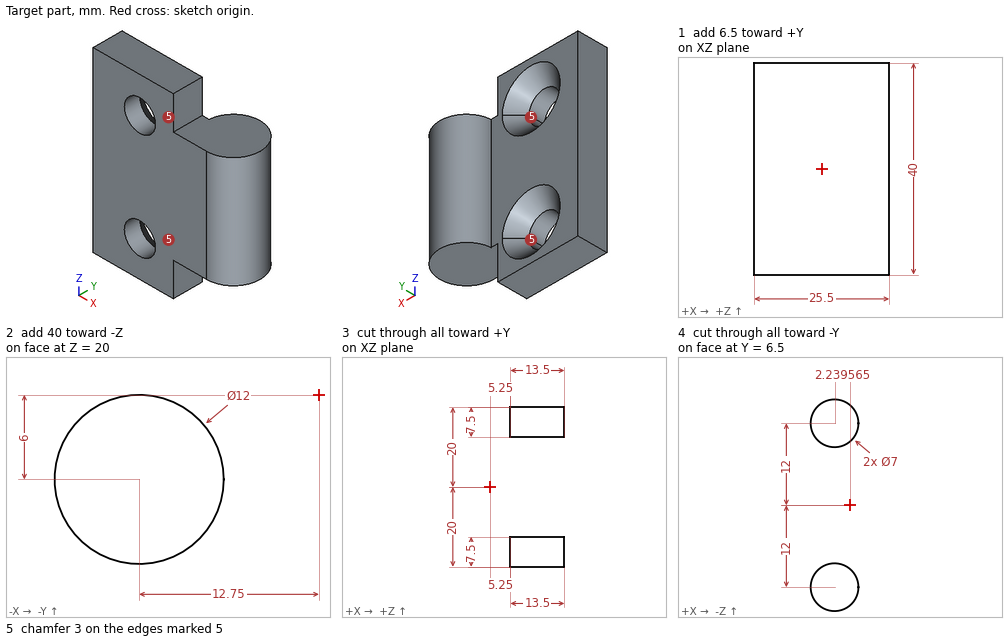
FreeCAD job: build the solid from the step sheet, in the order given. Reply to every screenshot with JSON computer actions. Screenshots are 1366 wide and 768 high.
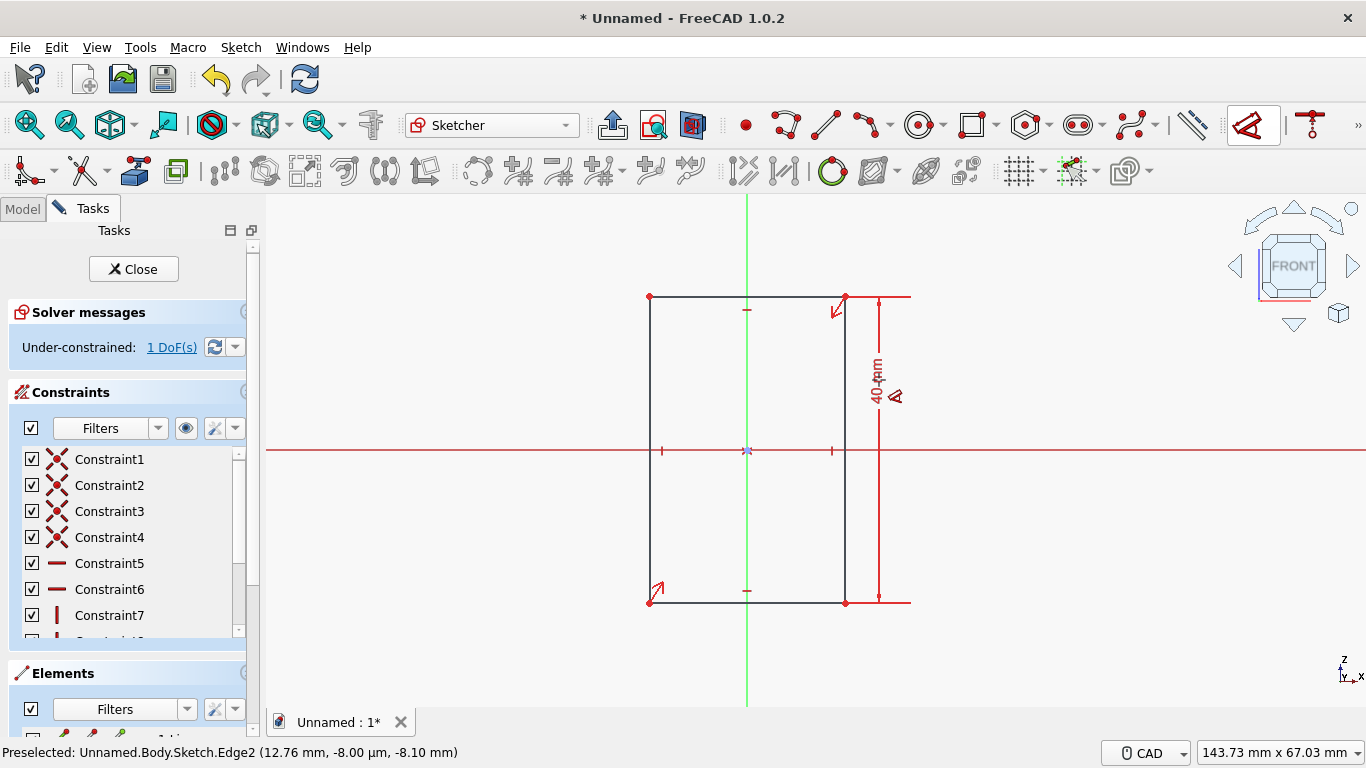
{"action": "left_click", "coordinate": [708, 603]}
{"action": "left_click", "coordinate": [702, 637]}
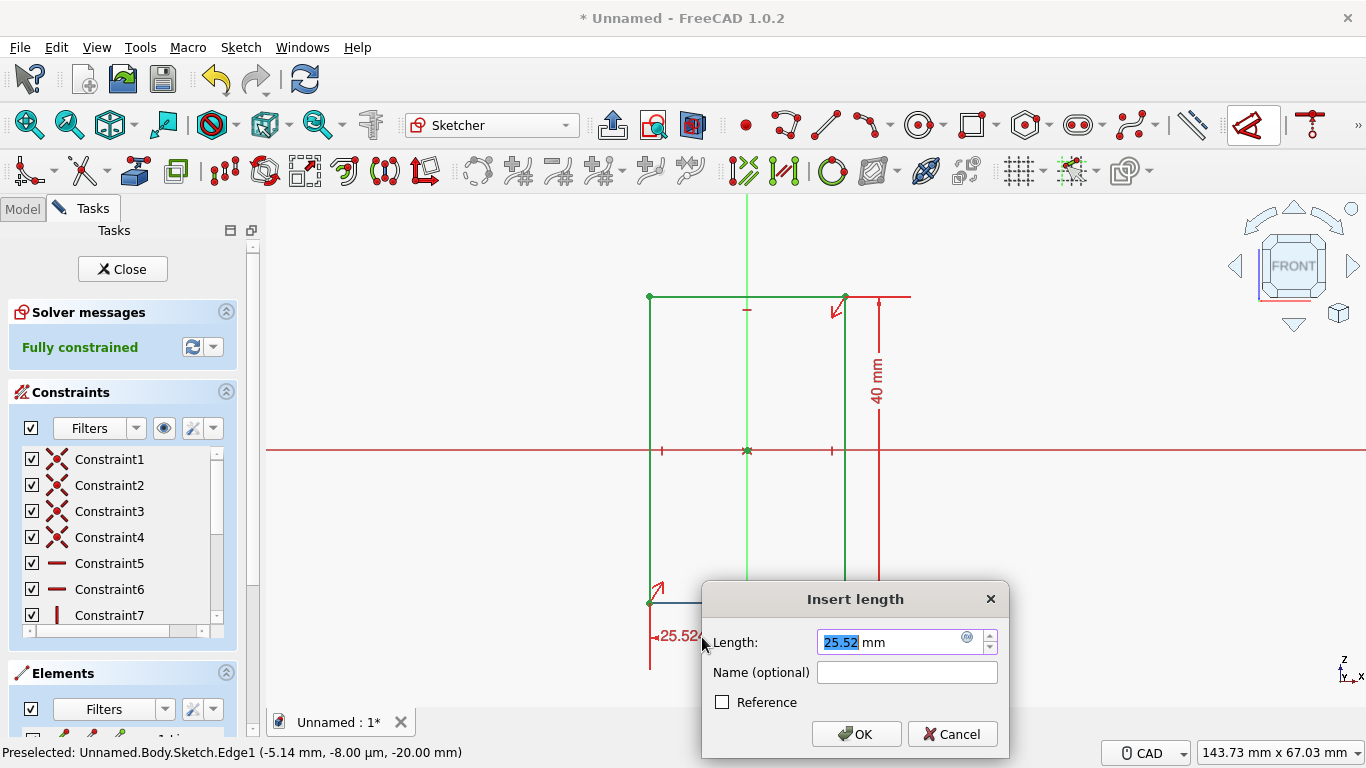
{"action": "type", "text": "25.5"}
{"action": "key", "text": "Return"}
{"action": "key", "text": "Escape"}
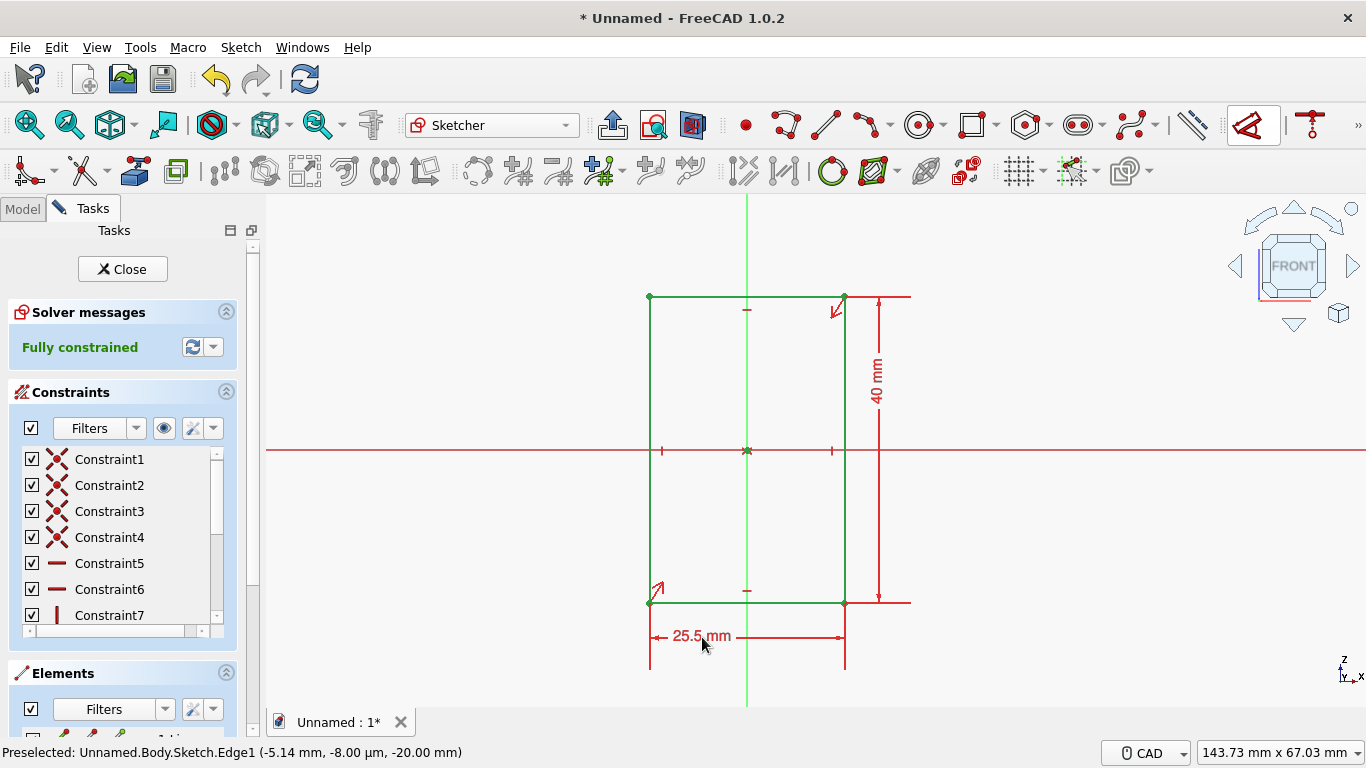
{"action": "left_click", "coordinate": [123, 269]}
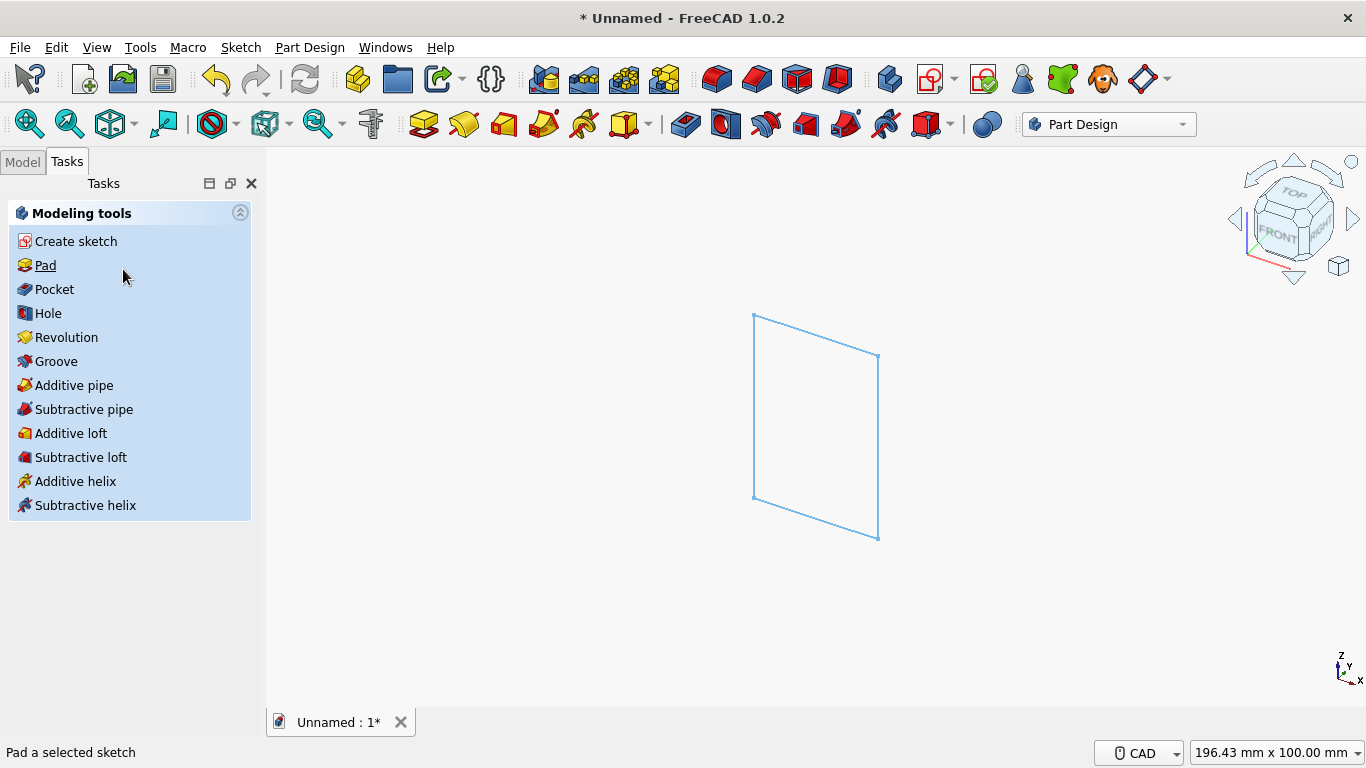
{"action": "left_click", "coordinate": [424, 124]}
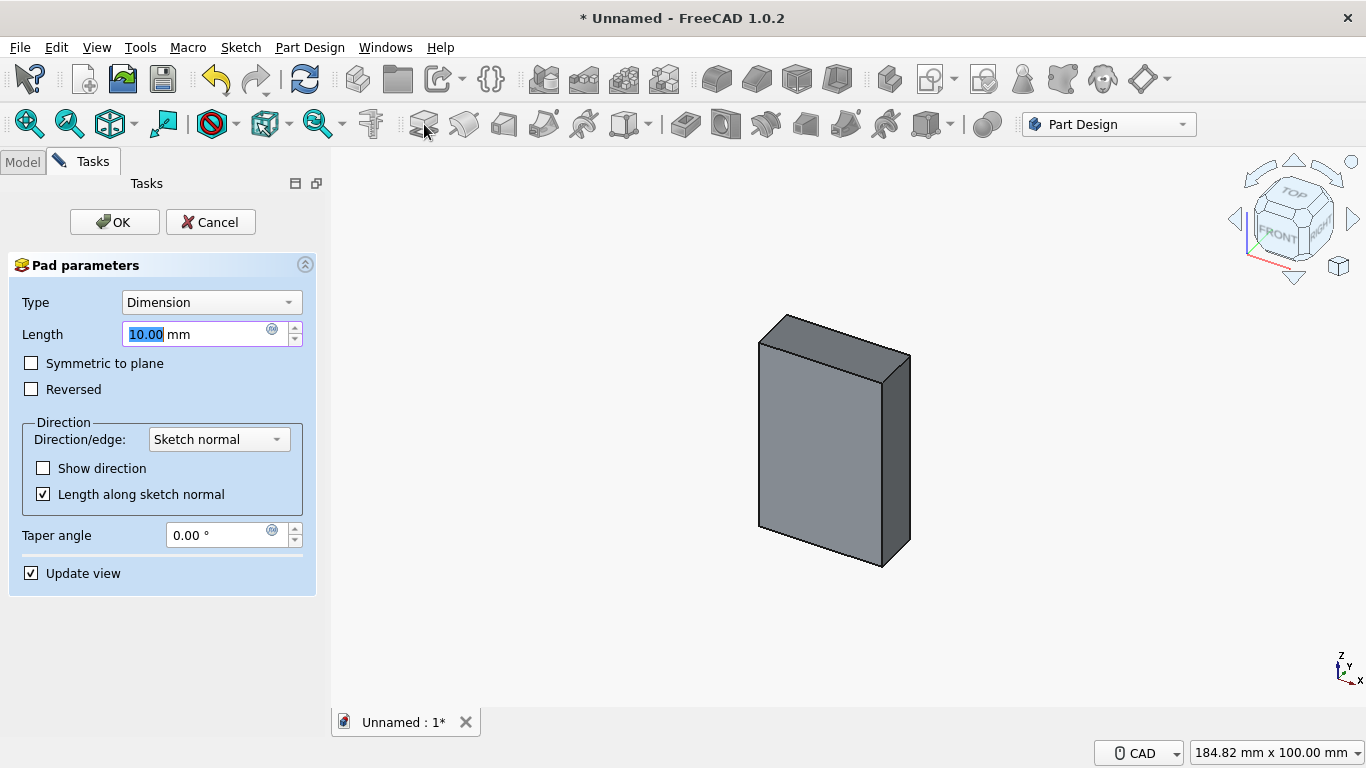
{"action": "type", "text": "6.5"}
{"action": "key", "text": "Tab"}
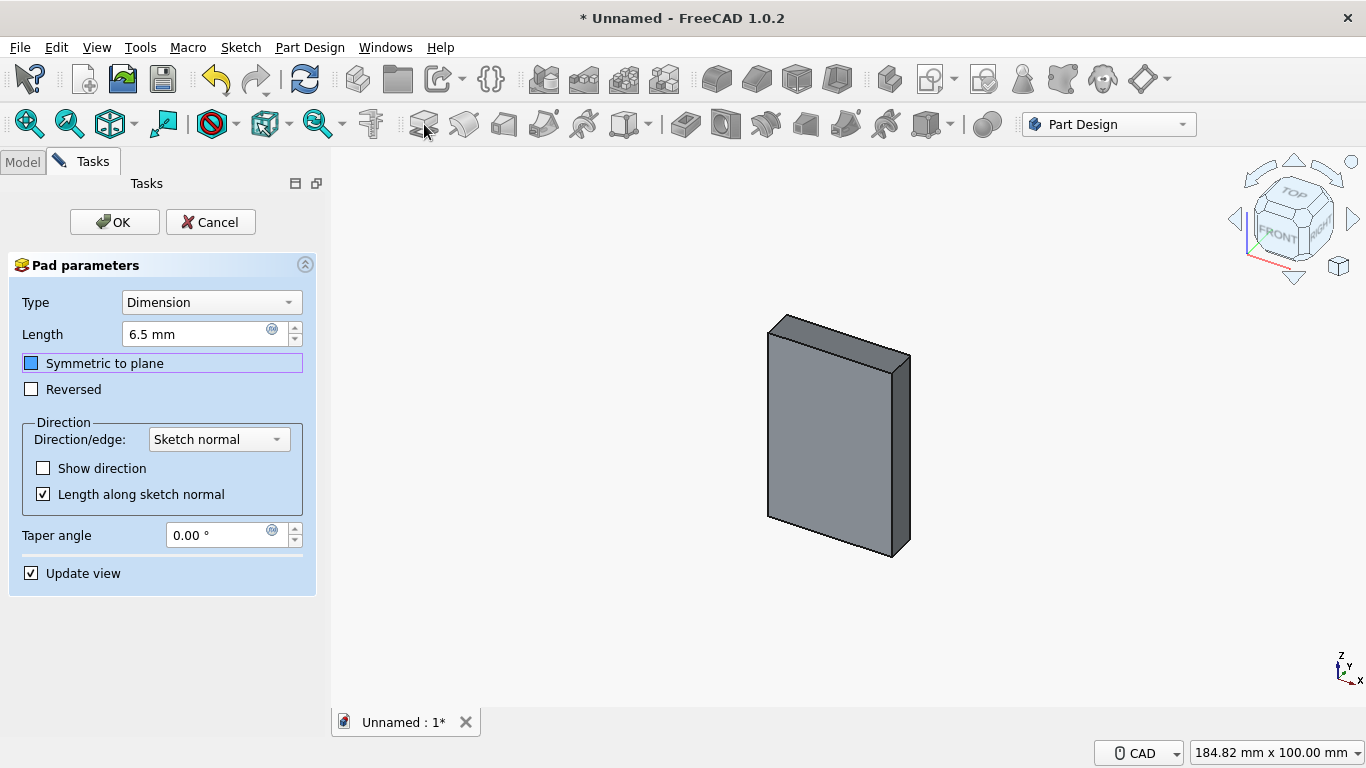
{"action": "left_click", "coordinate": [30, 389]}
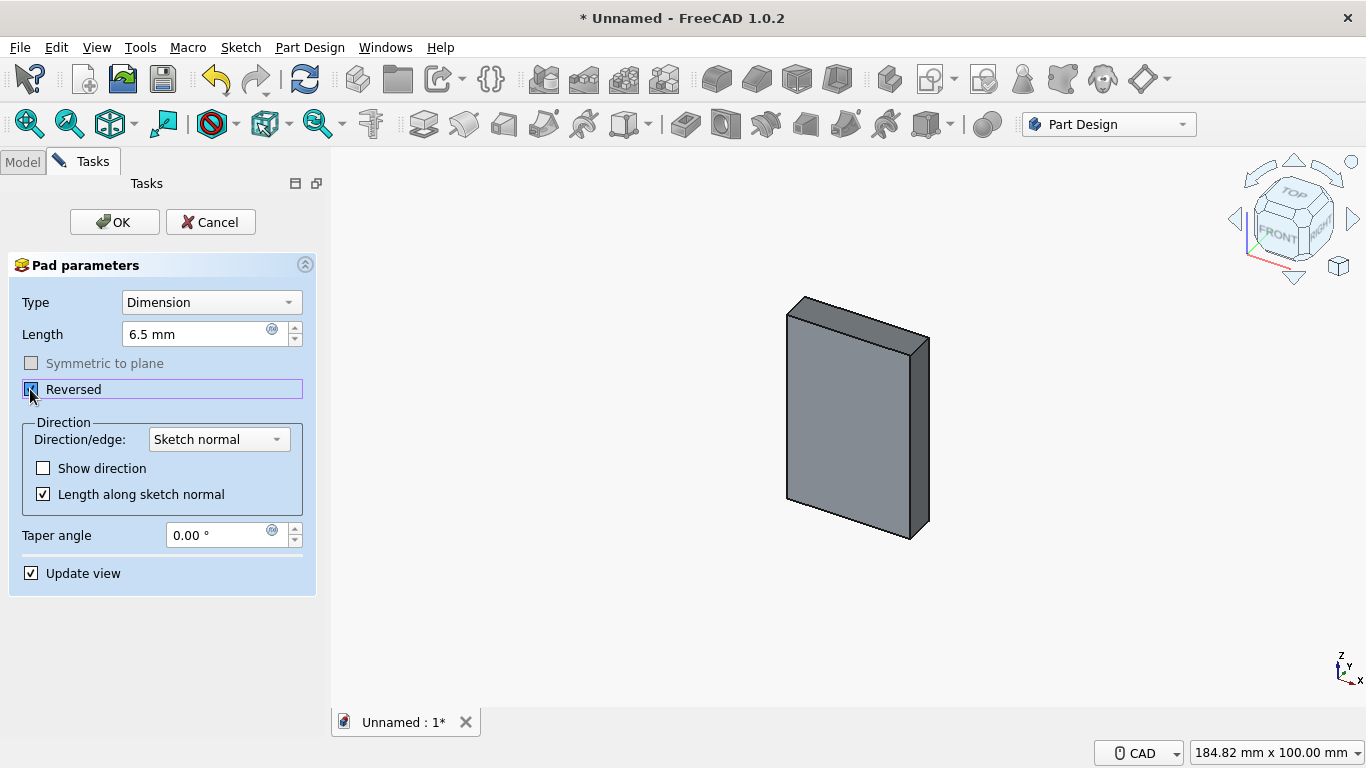
{"action": "left_click", "coordinate": [115, 222]}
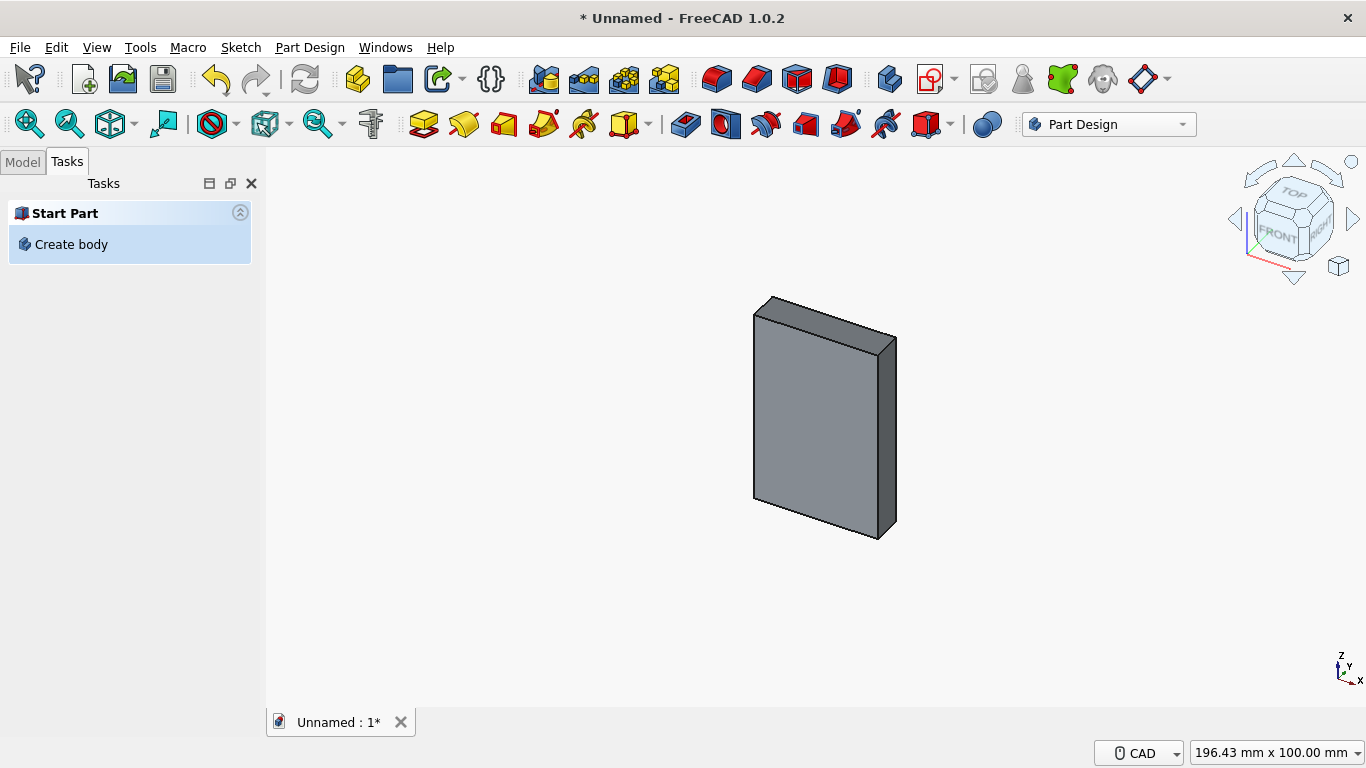
{"action": "key", "text": "v f"}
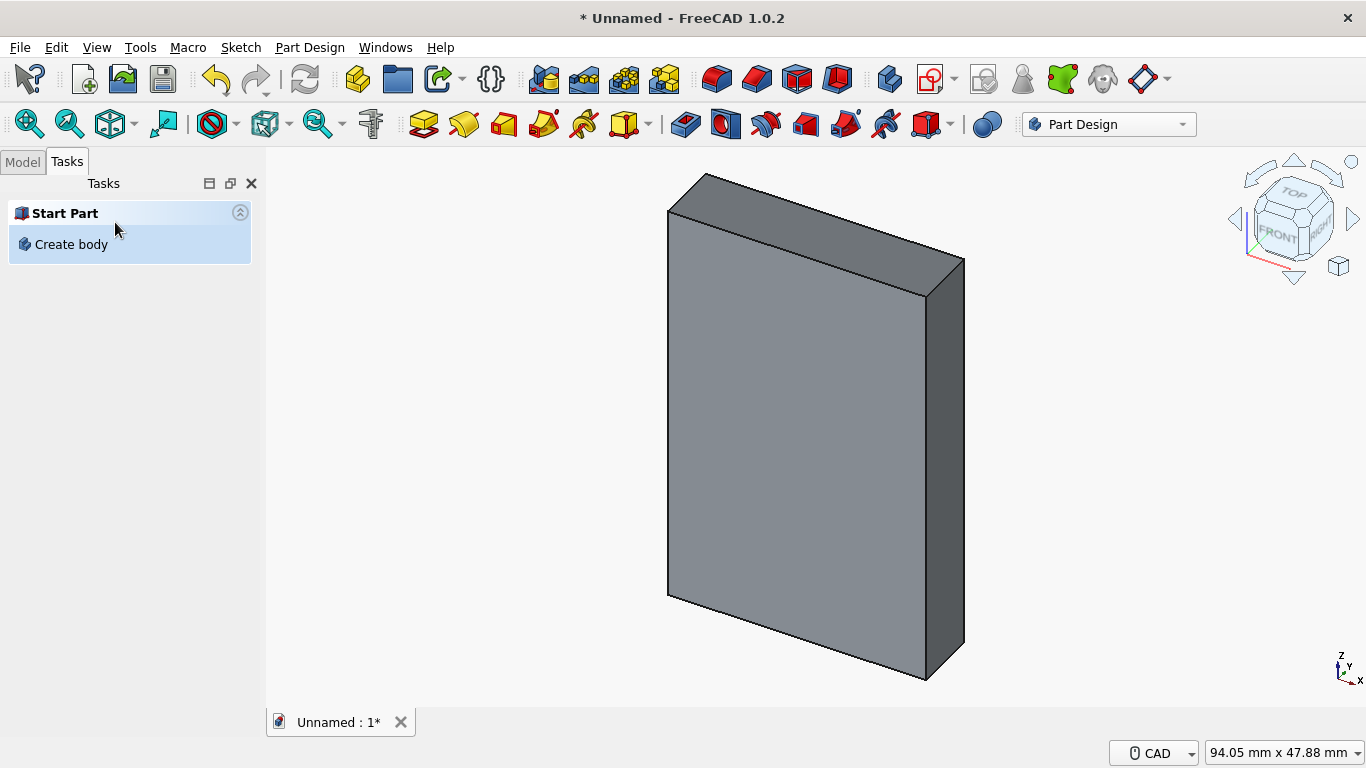
{"action": "left_click", "coordinate": [890, 259]}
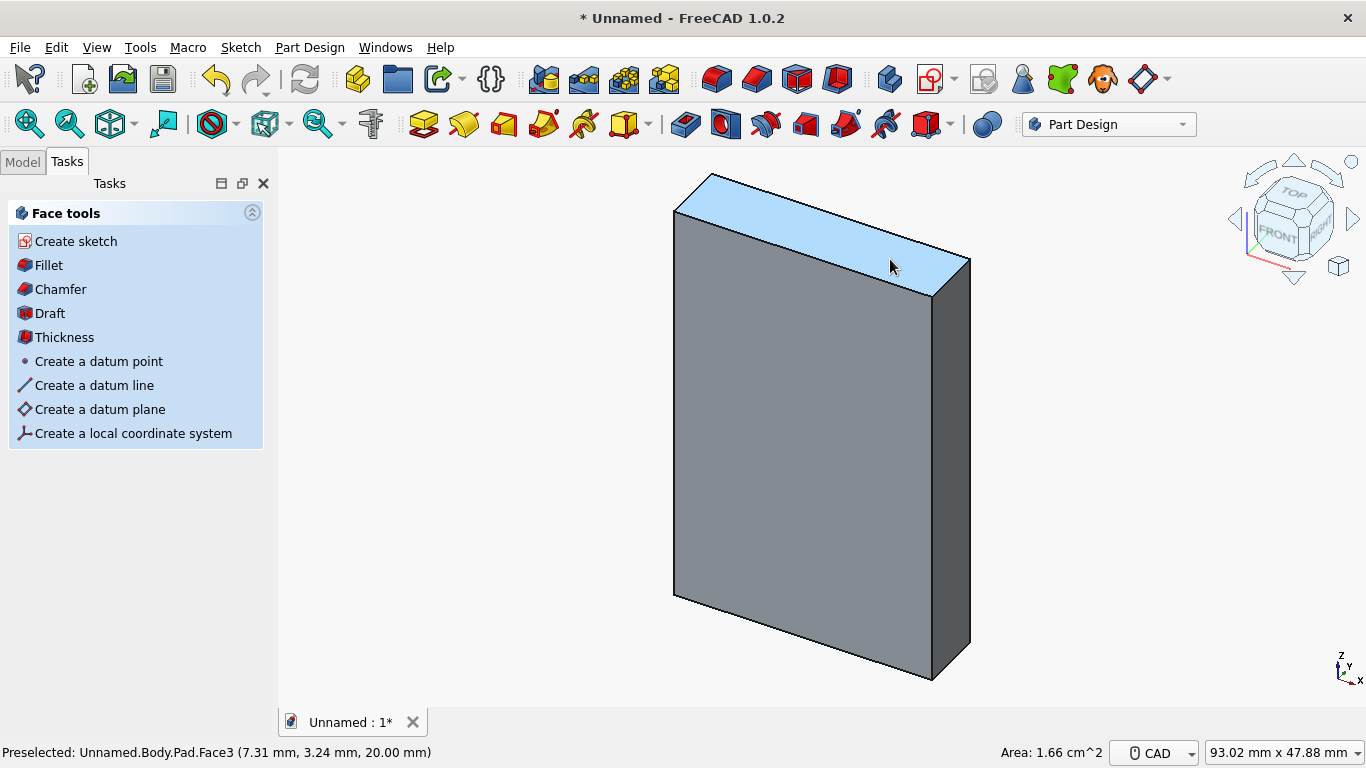
{"action": "left_click", "coordinate": [930, 80]}